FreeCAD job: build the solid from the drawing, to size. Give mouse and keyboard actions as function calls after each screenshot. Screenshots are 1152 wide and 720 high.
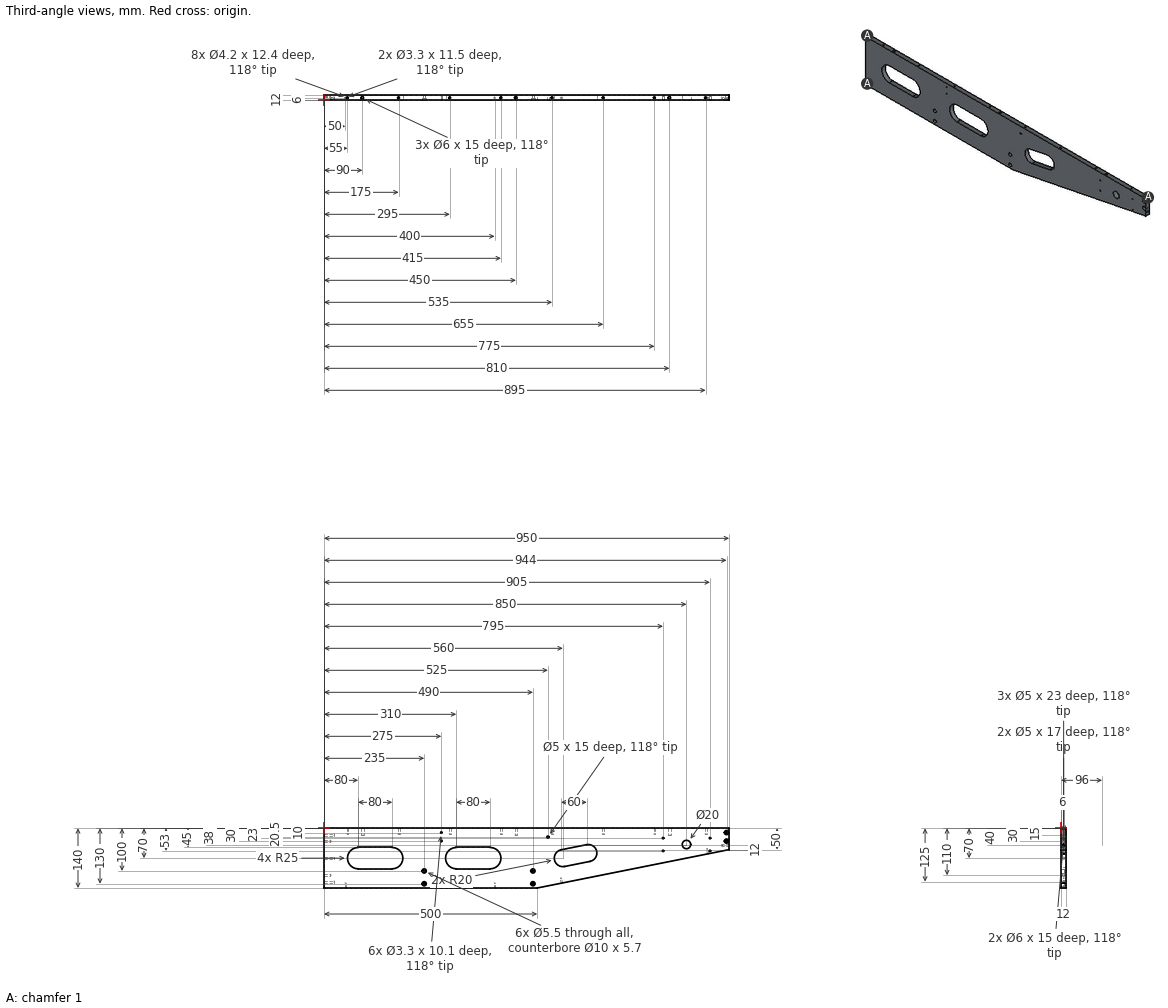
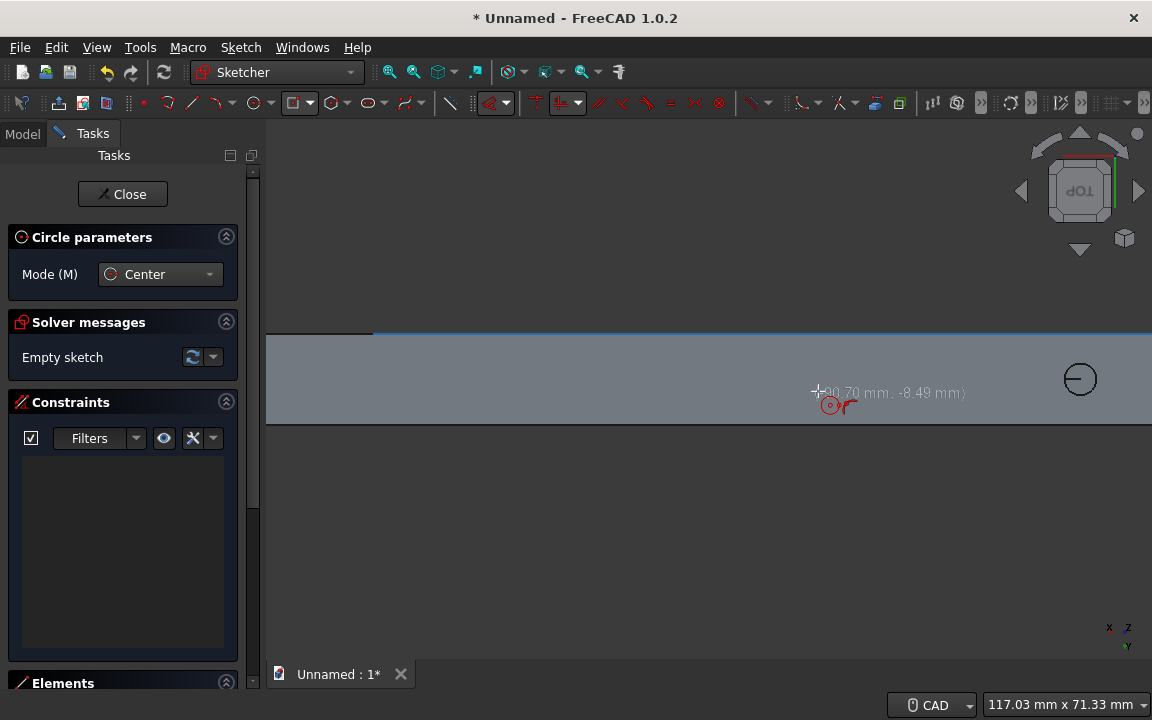
click(816, 379)
move(832, 363)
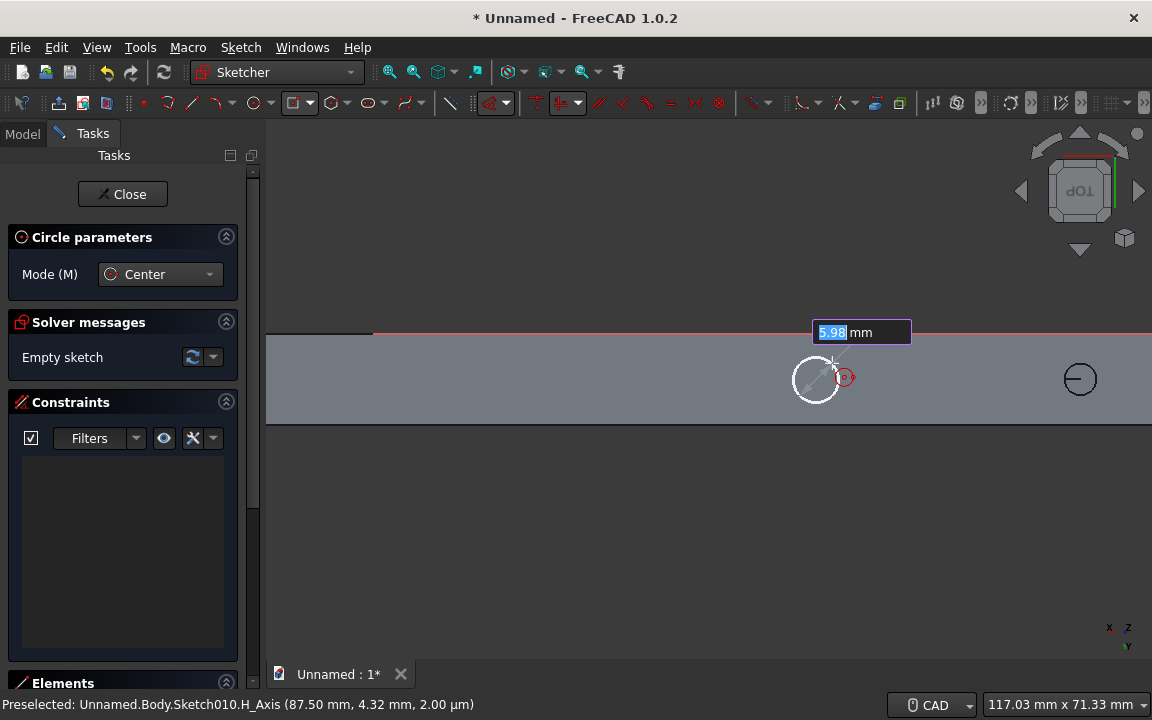
text(6)
key(Return)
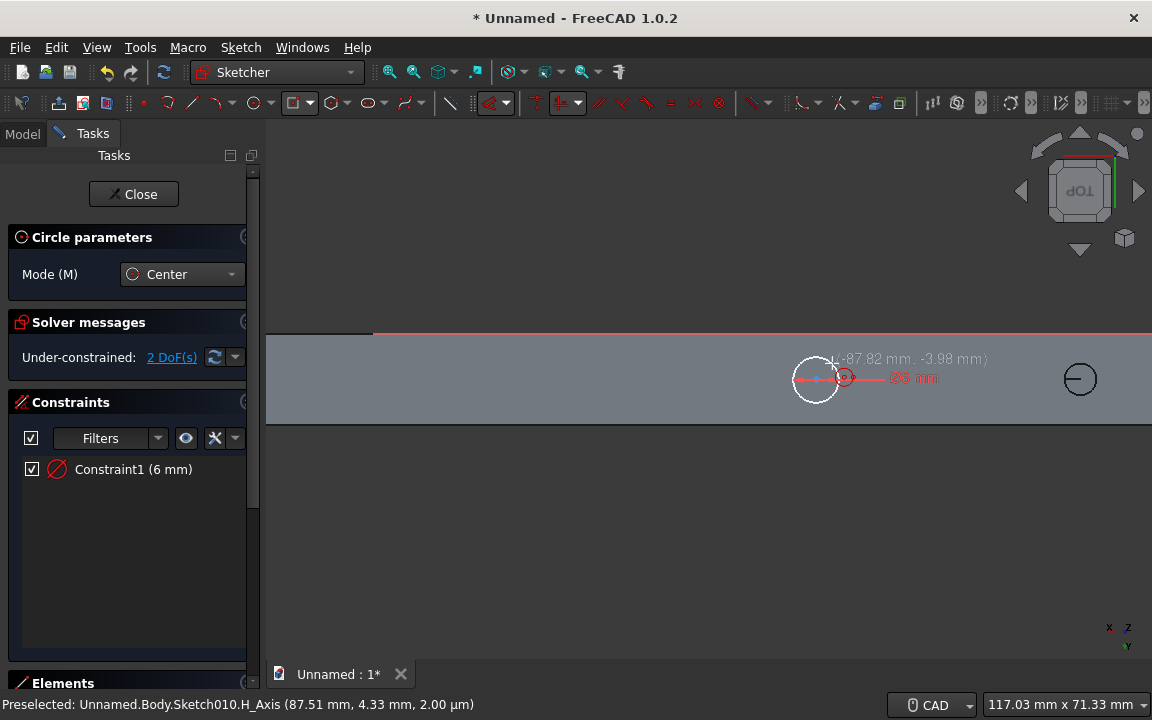
scroll(819, 391, down, 13)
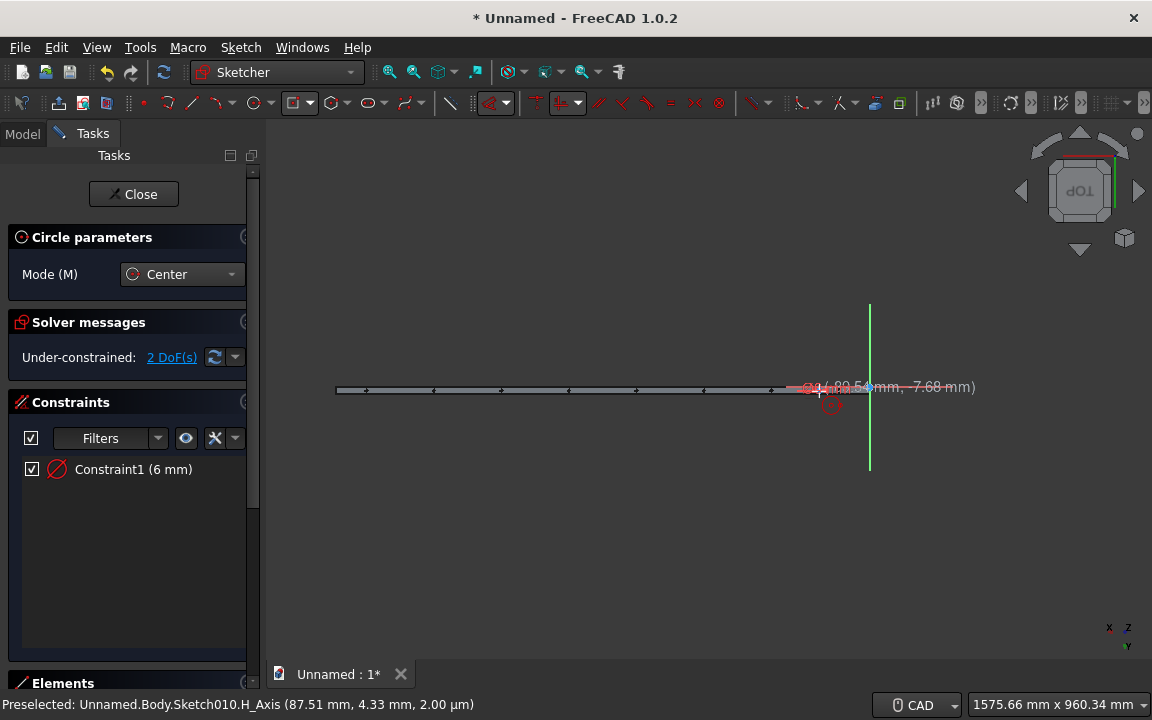
scroll(617, 391, up, 13)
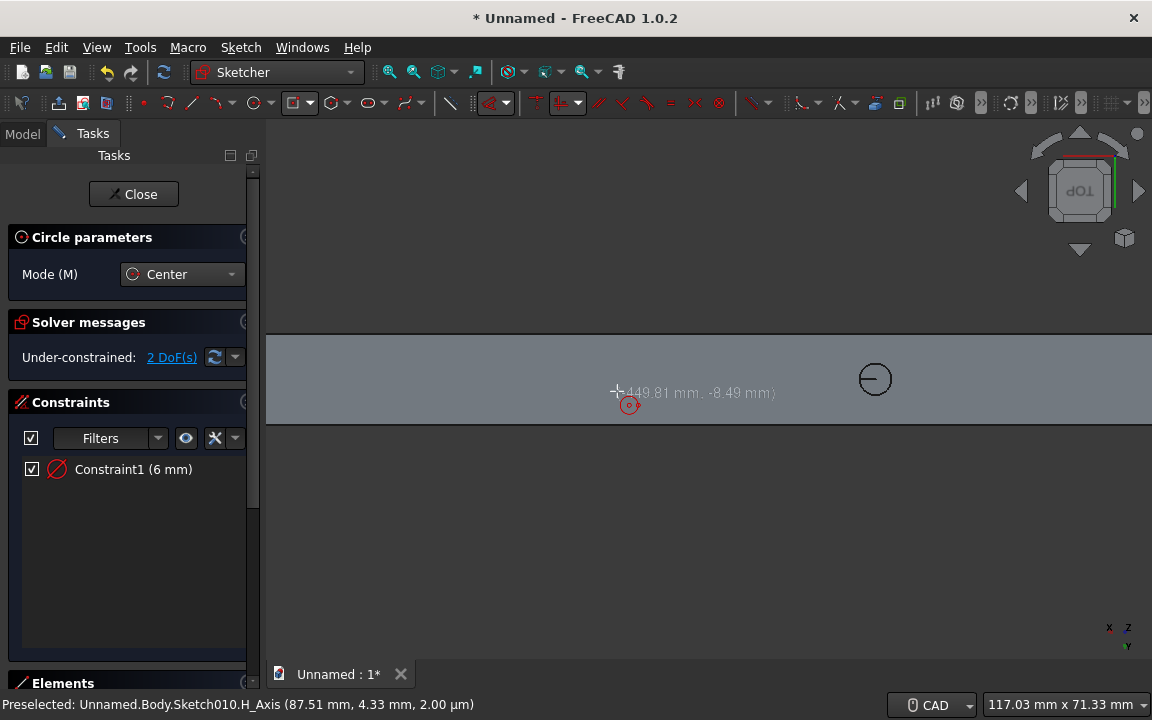
click(611, 379)
move(627, 363)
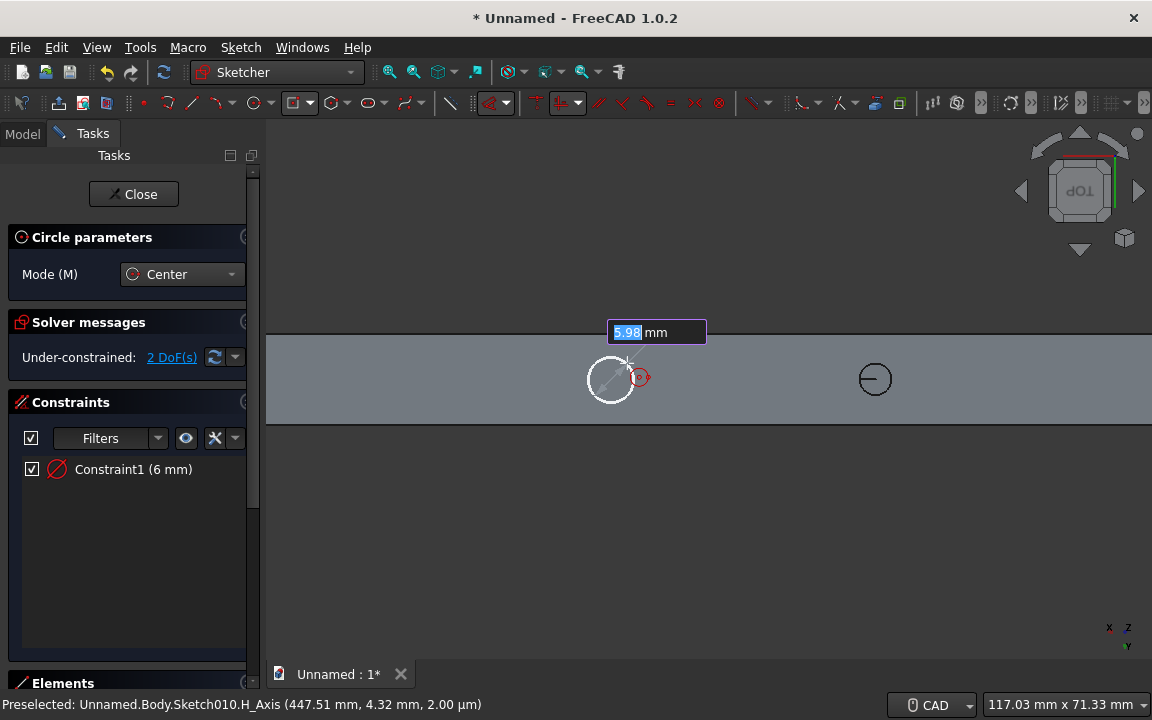
text(6)
key(Return)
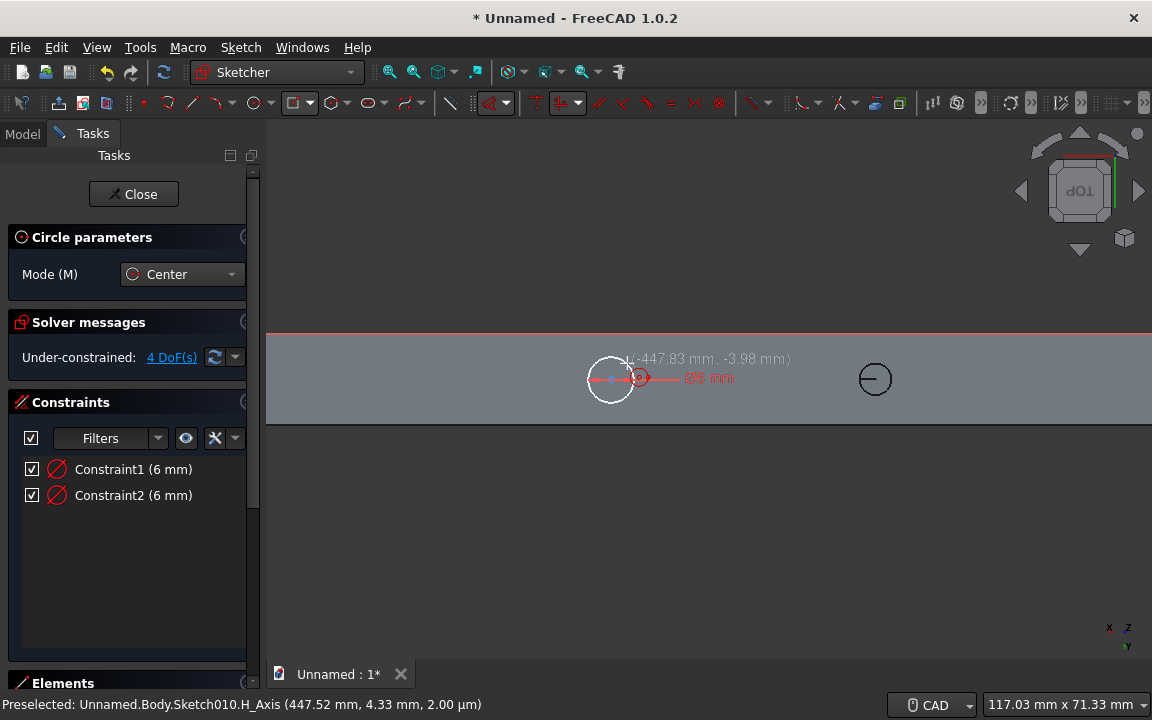
scroll(616, 391, down, 13)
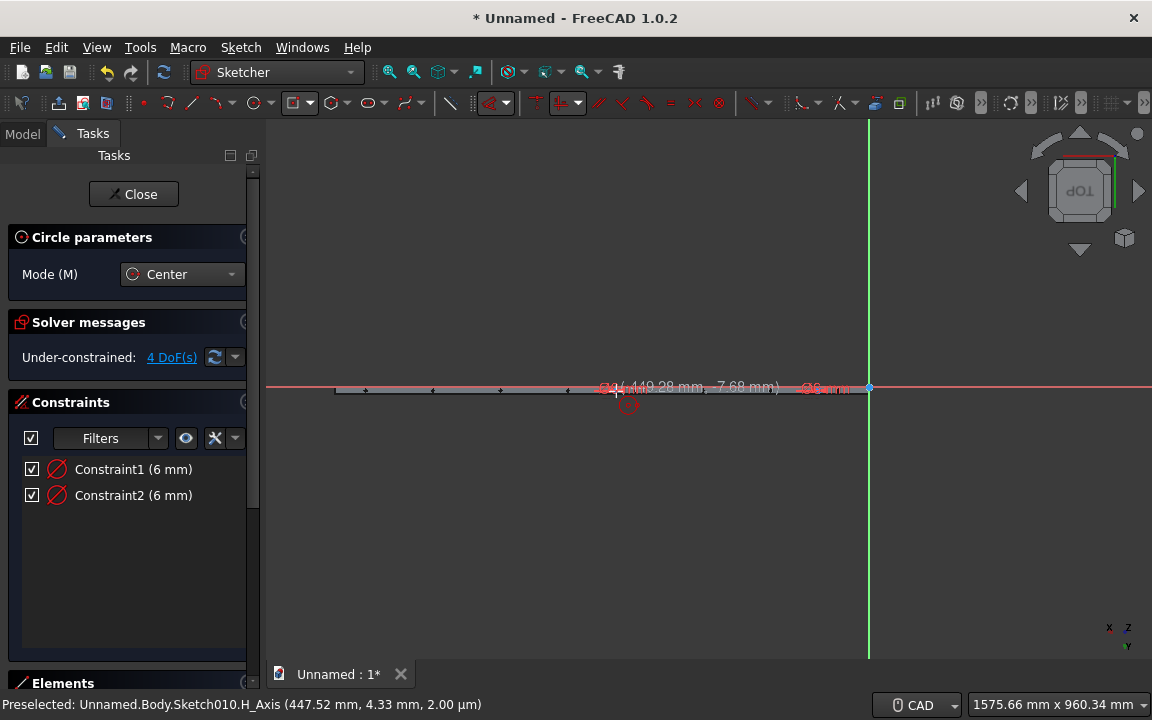
scroll(414, 391, up, 13)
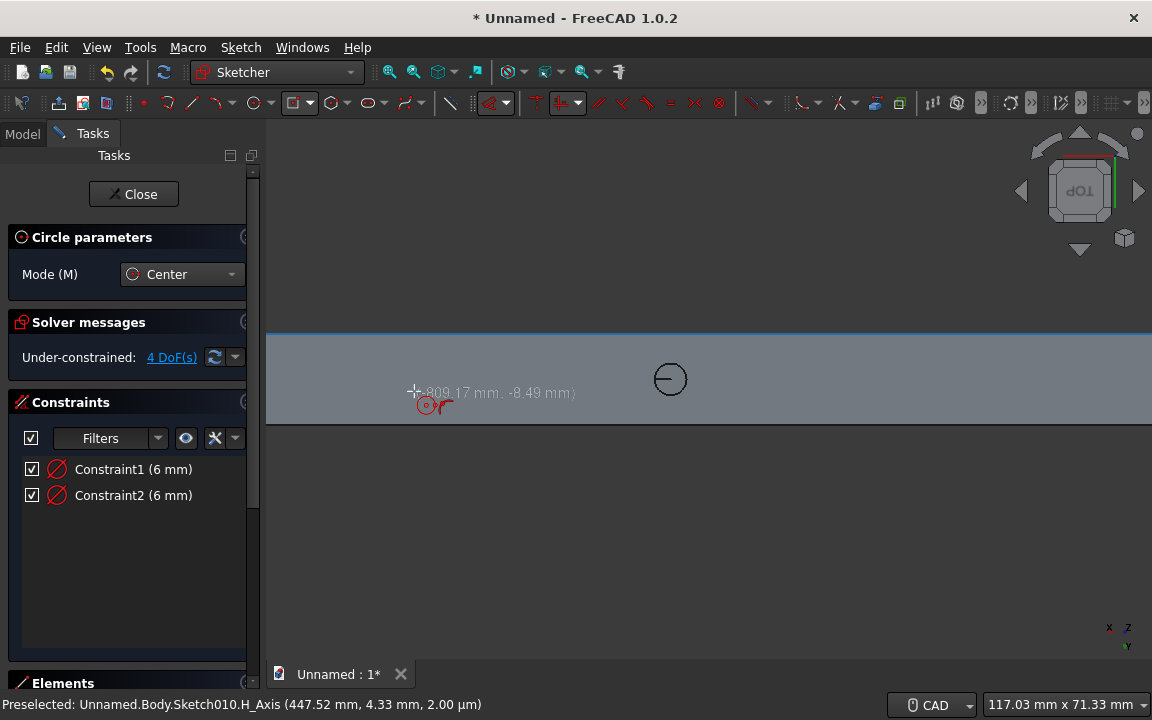
click(406, 379)
move(422, 363)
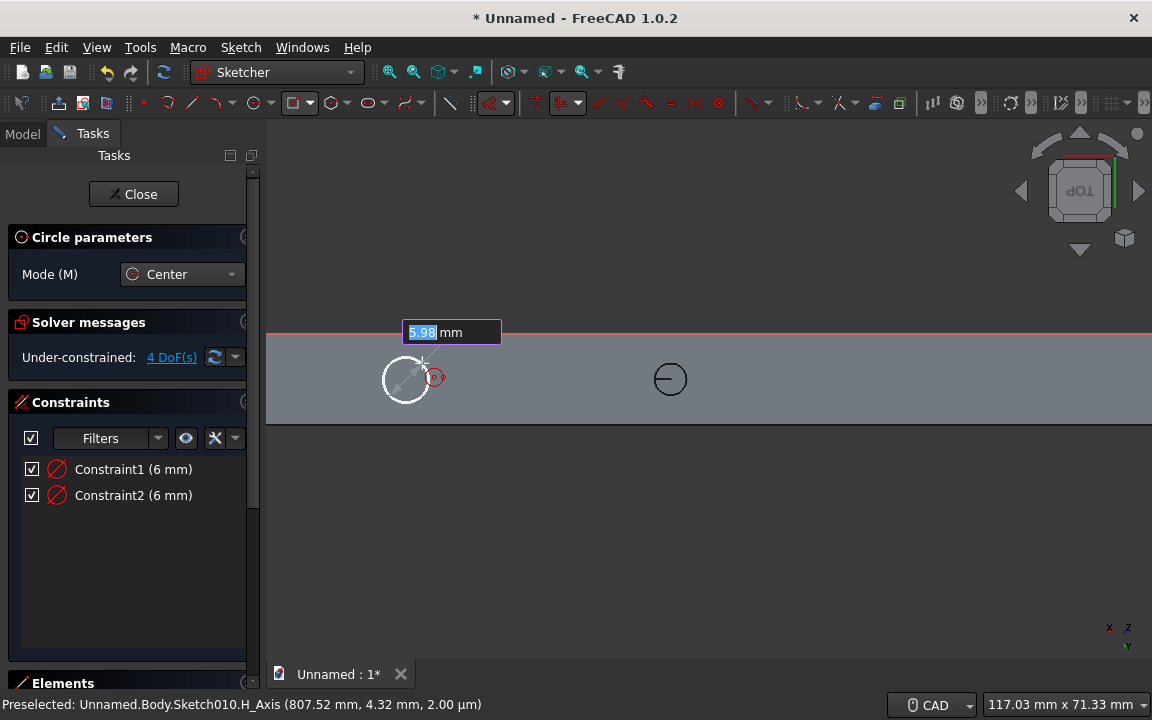
text(6)
key(Return)
key(Escape)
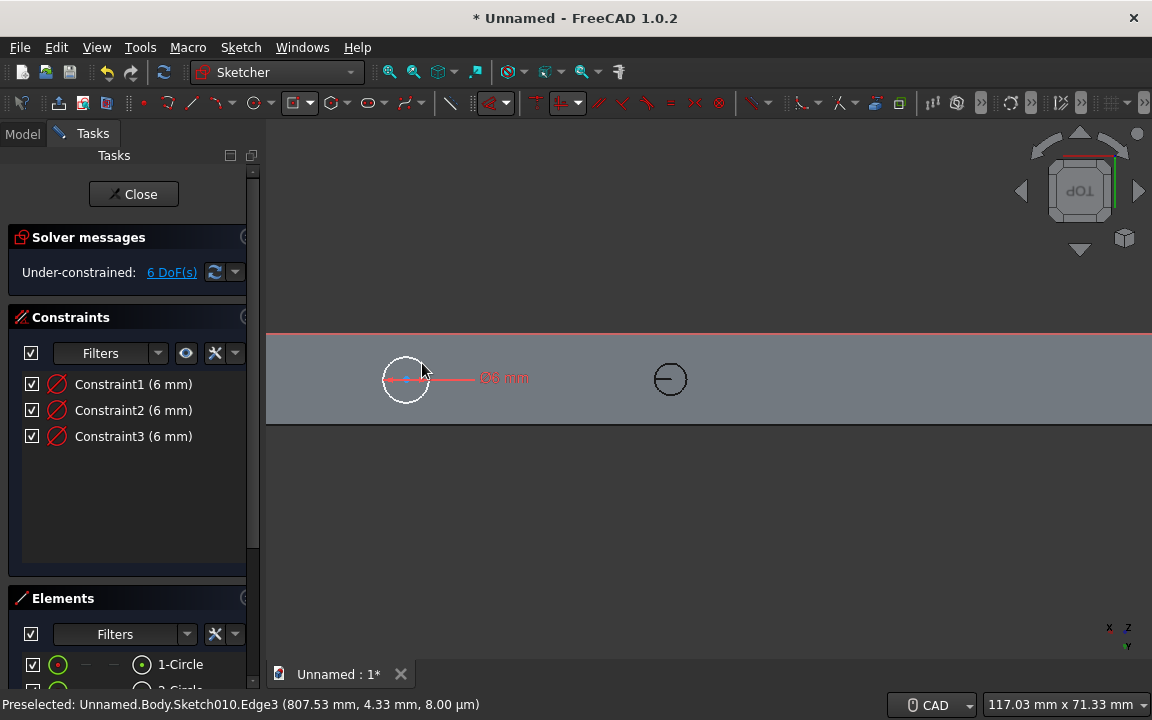
scroll(414, 391, down, 13)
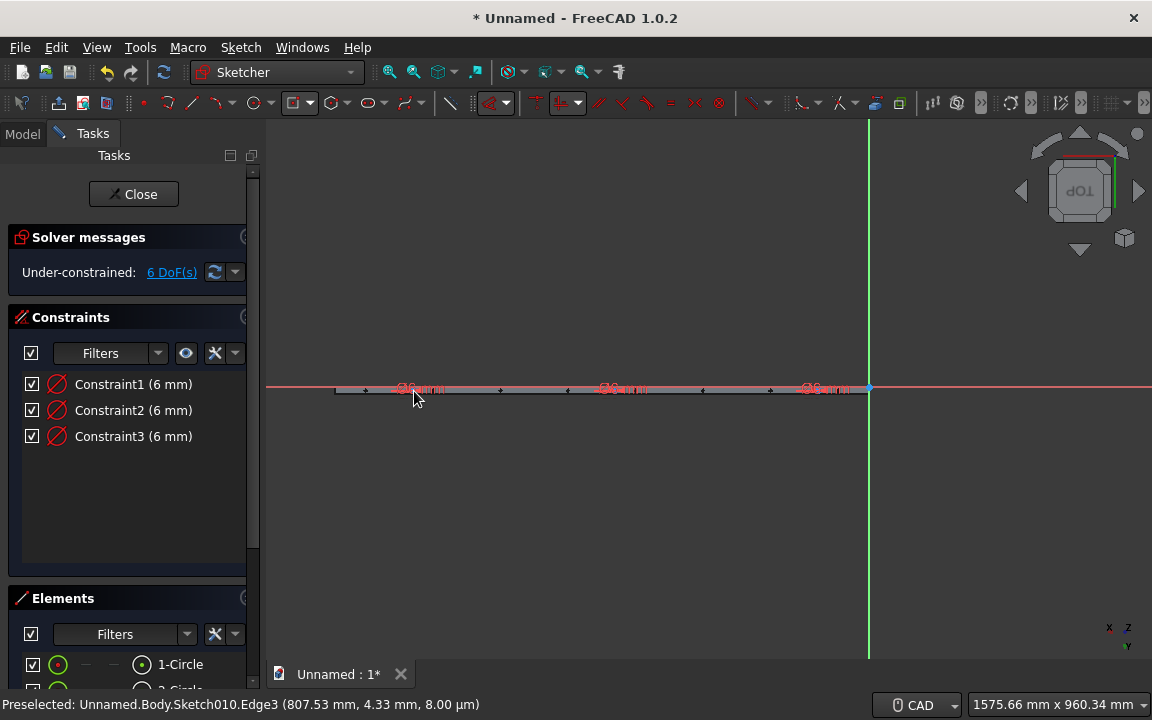
click(818, 391)